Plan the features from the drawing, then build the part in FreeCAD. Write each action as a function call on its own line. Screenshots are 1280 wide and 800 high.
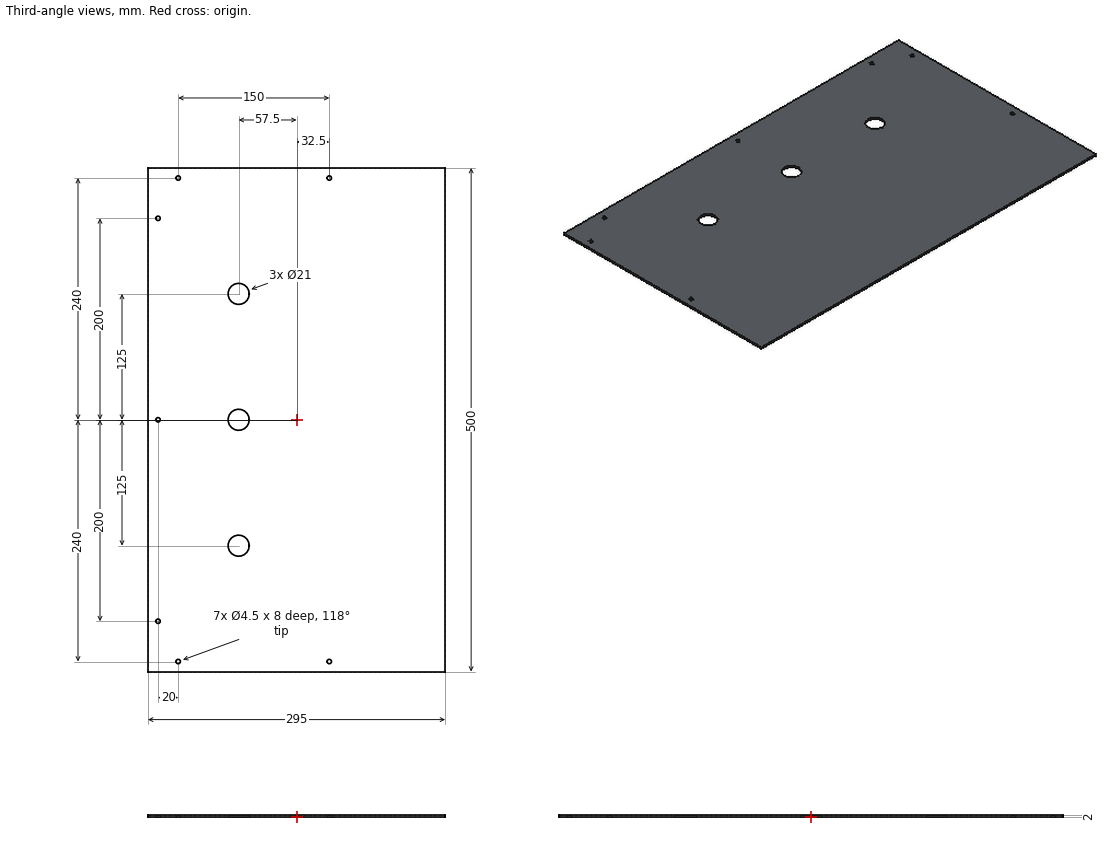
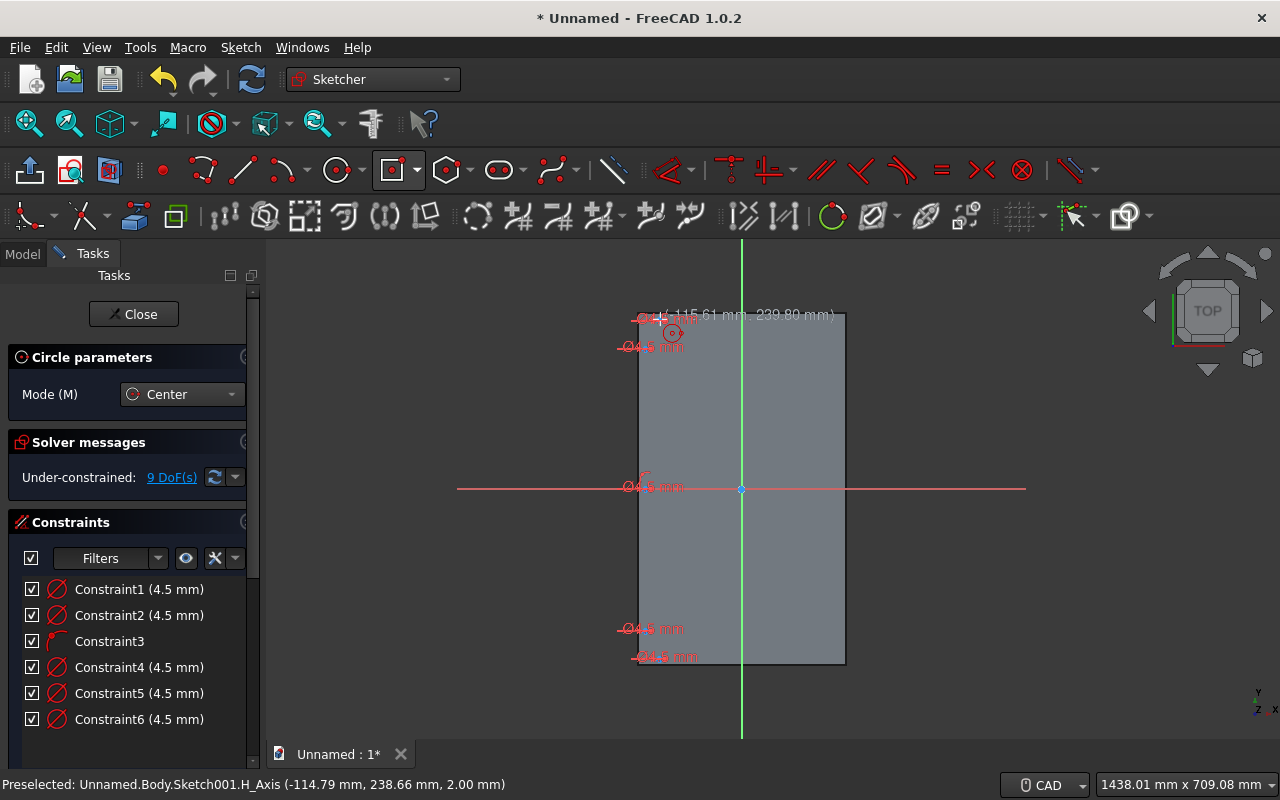
scroll(764, 320, up, 14)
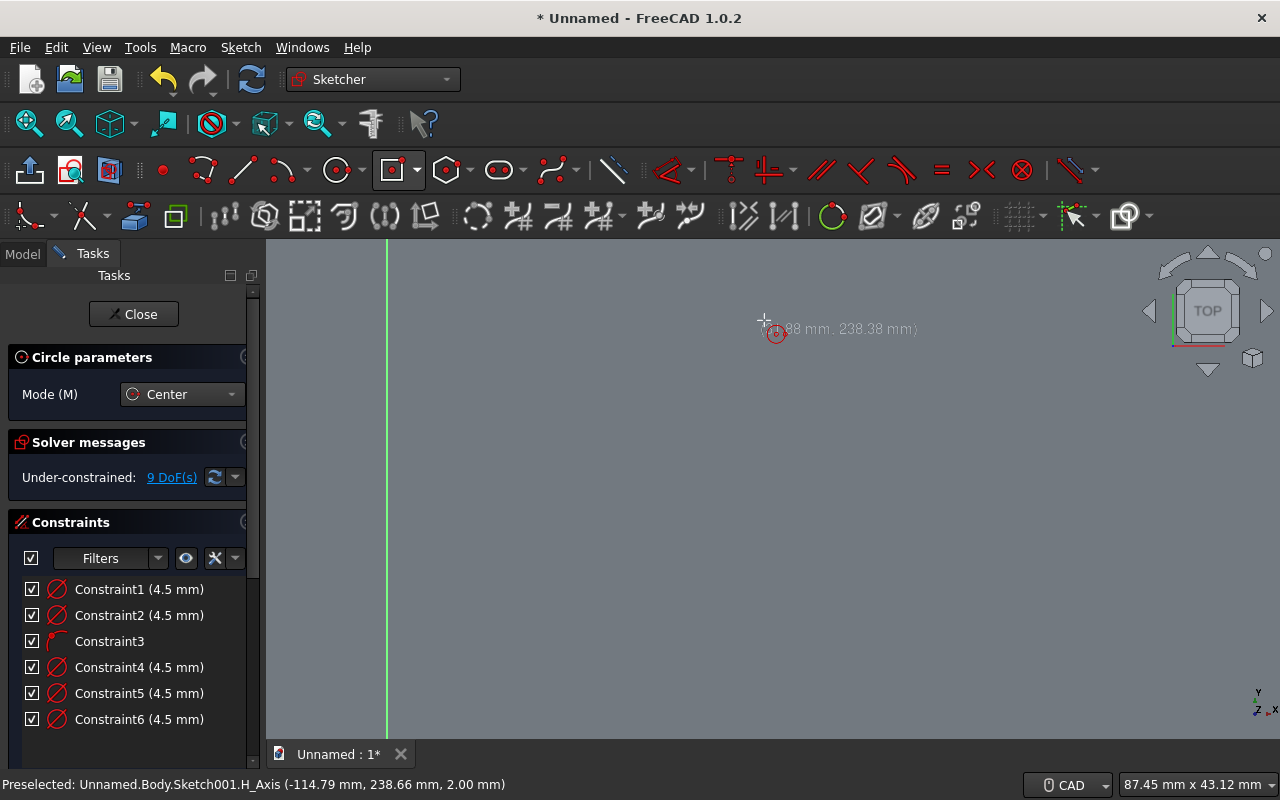
scroll(764, 320, down, 14)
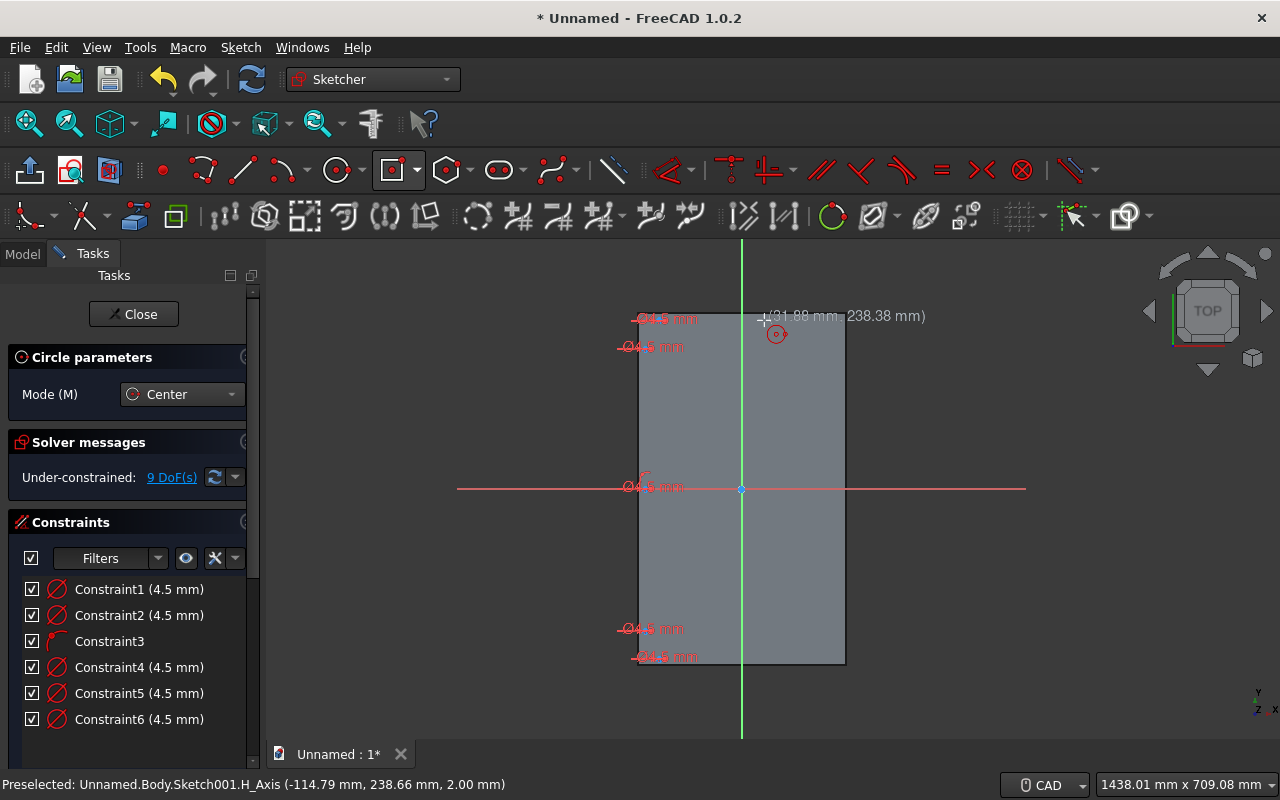
click(764, 320)
move(766, 319)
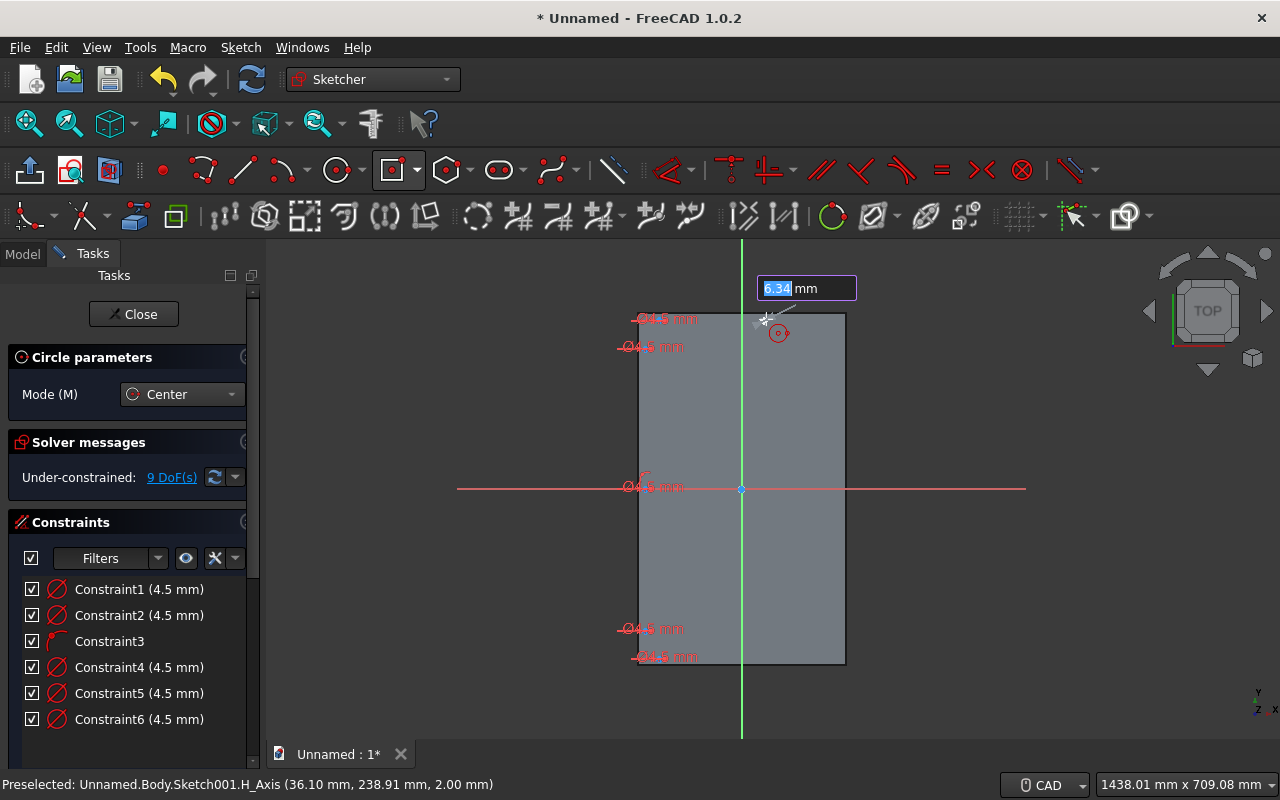
text(4.5)
key(Return)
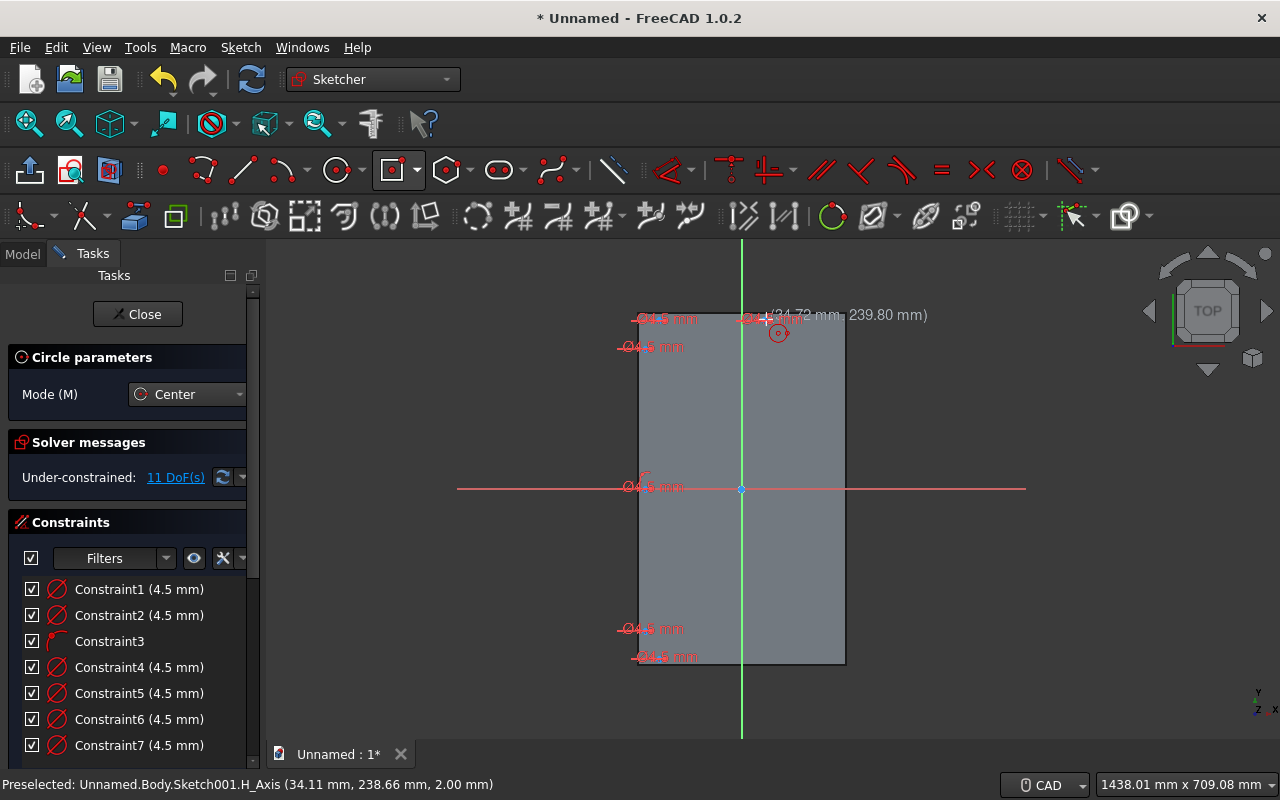
scroll(764, 658, up, 14)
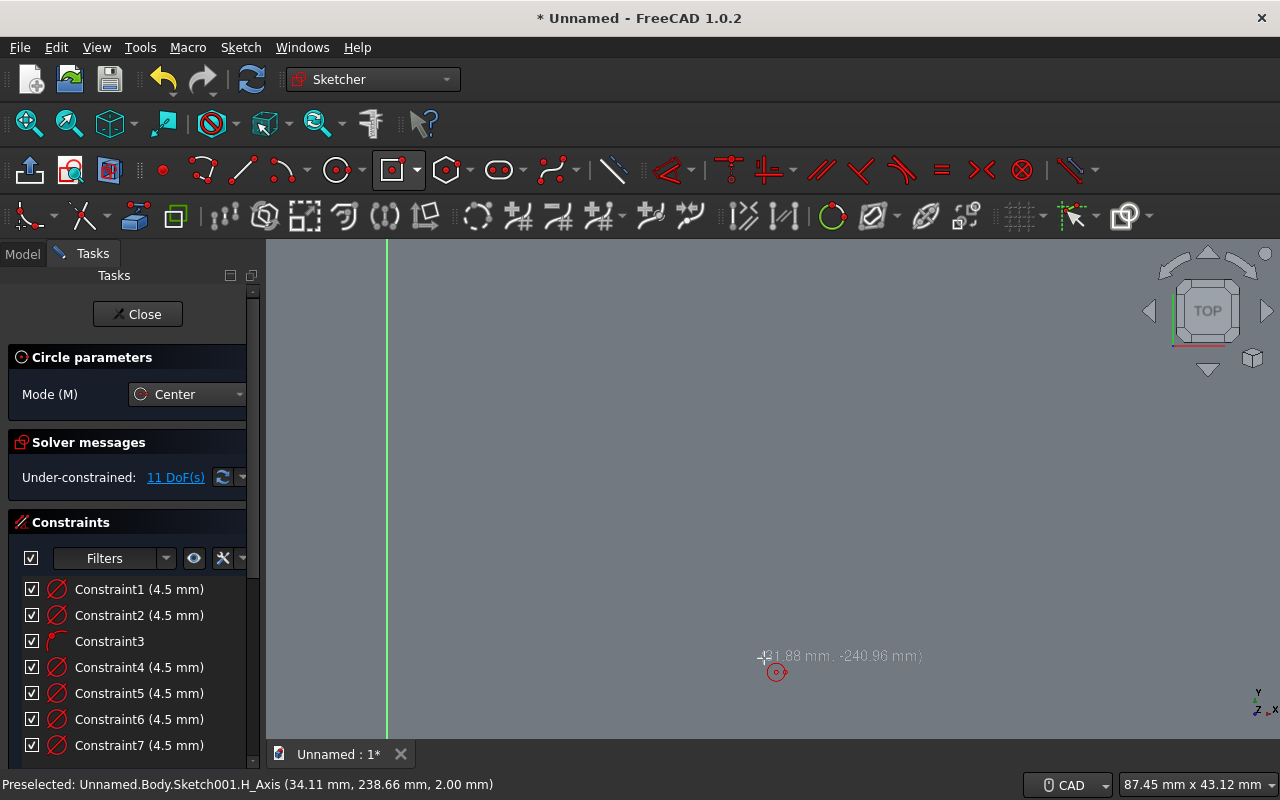
scroll(764, 659, down, 14)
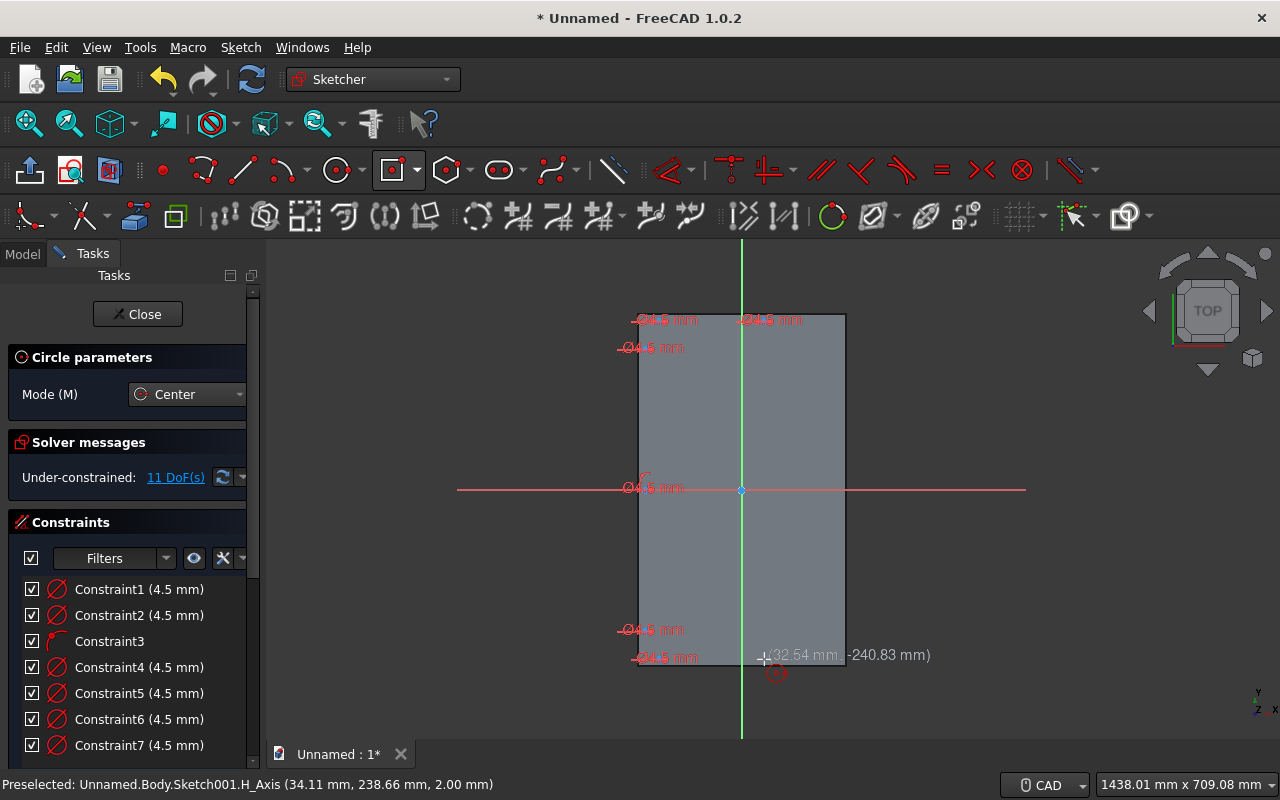
click(764, 659)
move(766, 658)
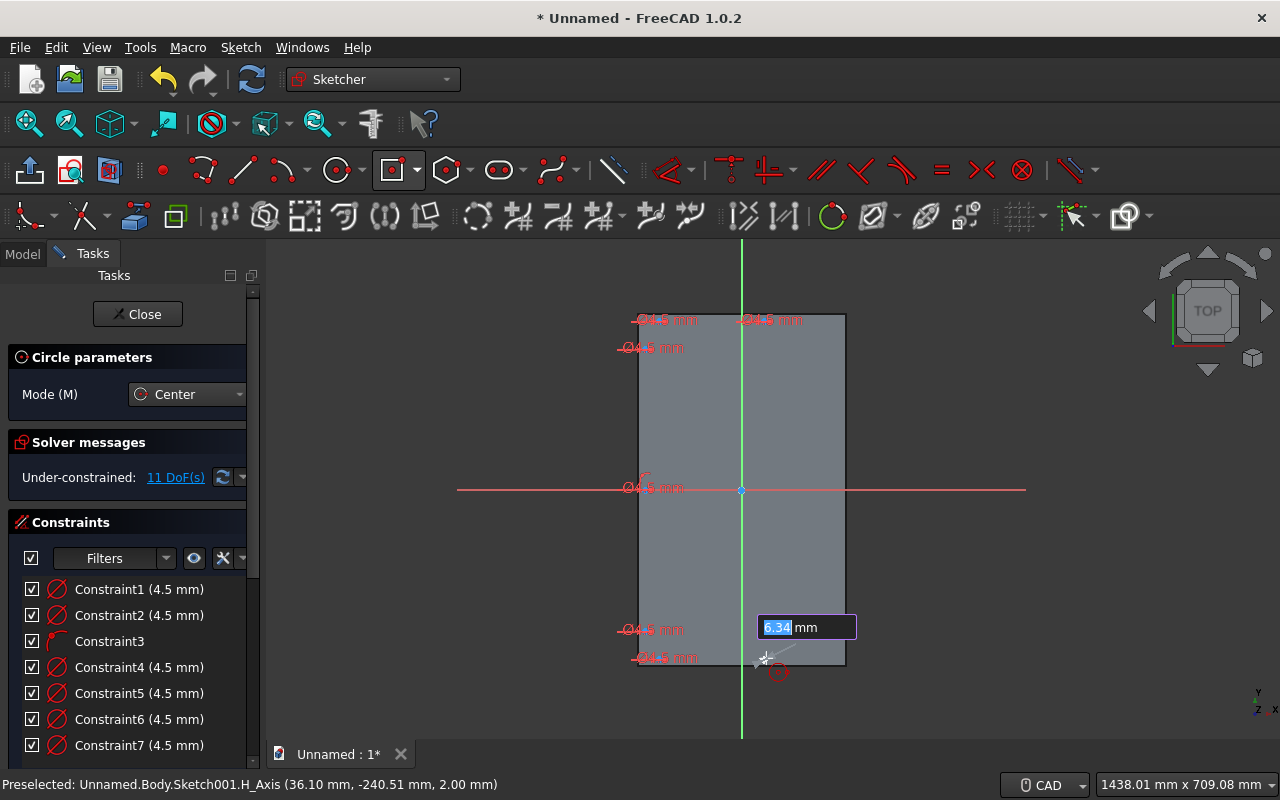
text(4.5)
key(Return)
key(Escape)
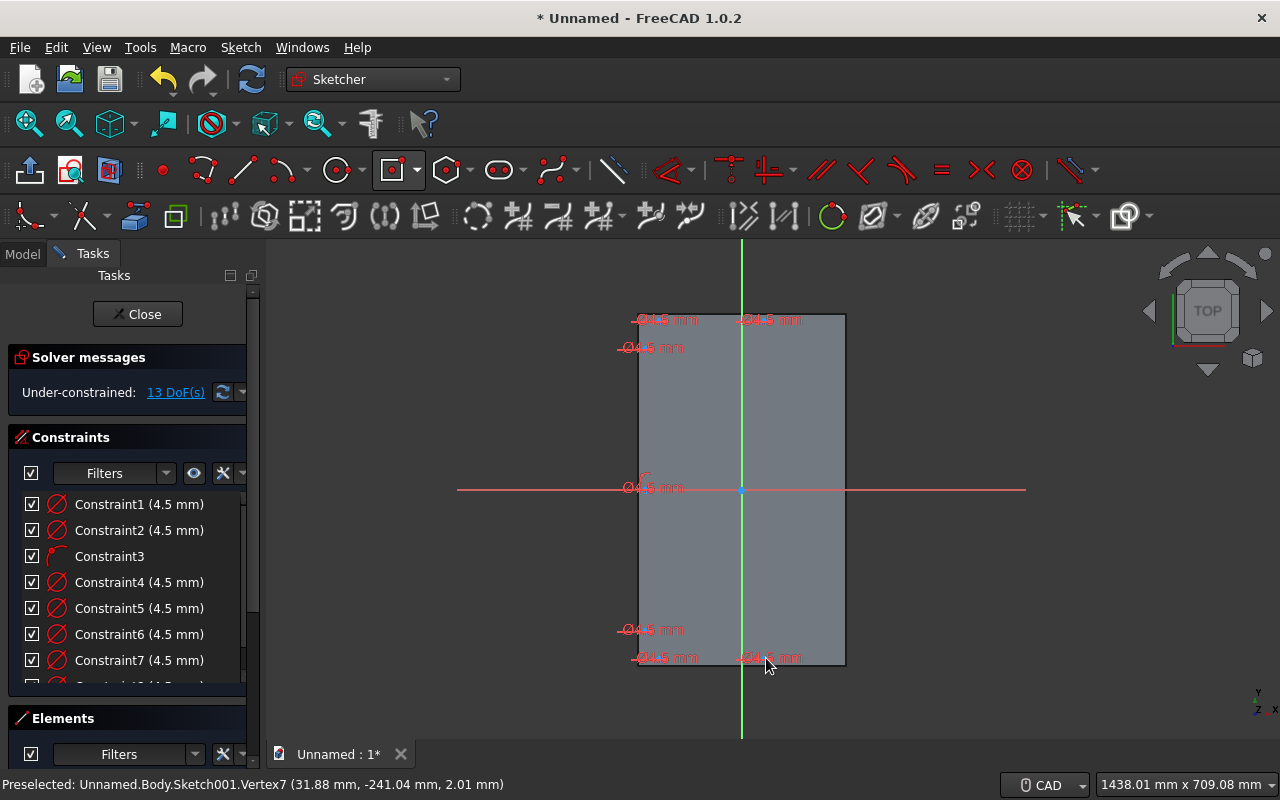
click(645, 490)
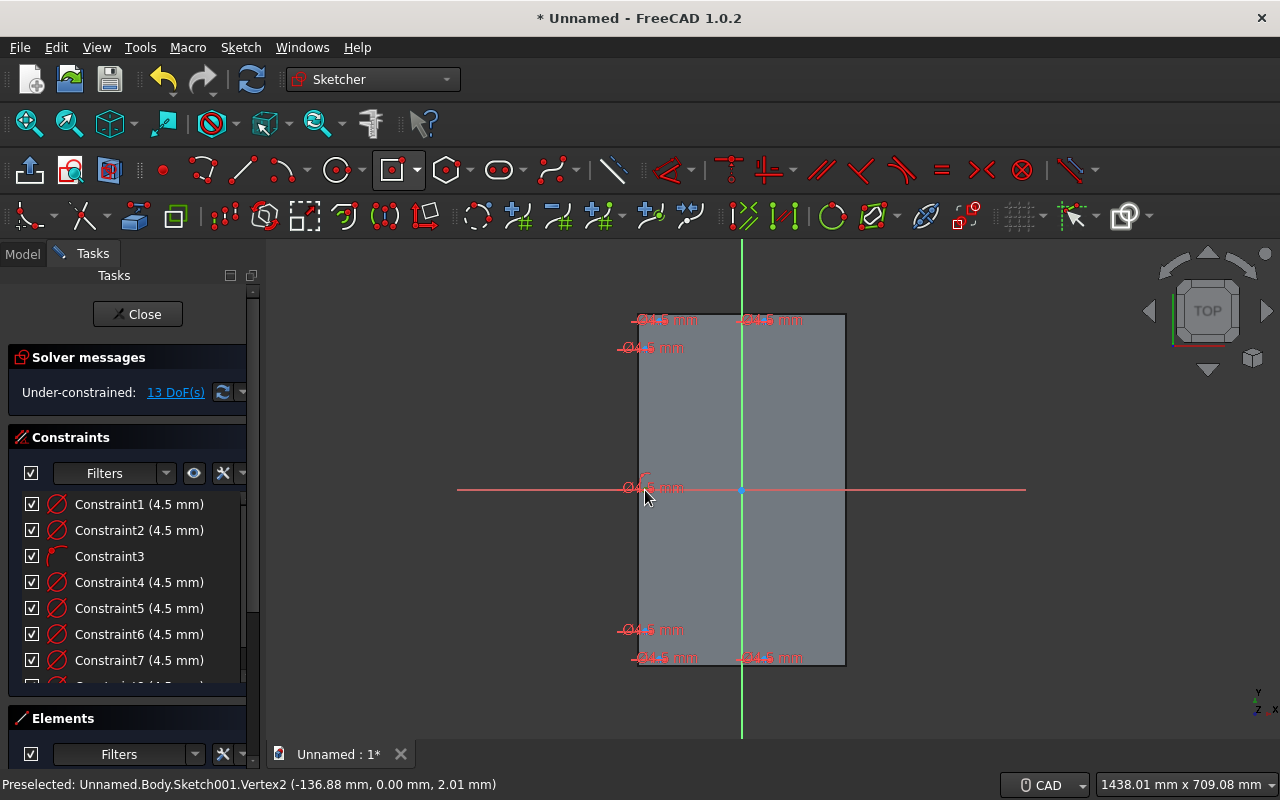
click(645, 350)